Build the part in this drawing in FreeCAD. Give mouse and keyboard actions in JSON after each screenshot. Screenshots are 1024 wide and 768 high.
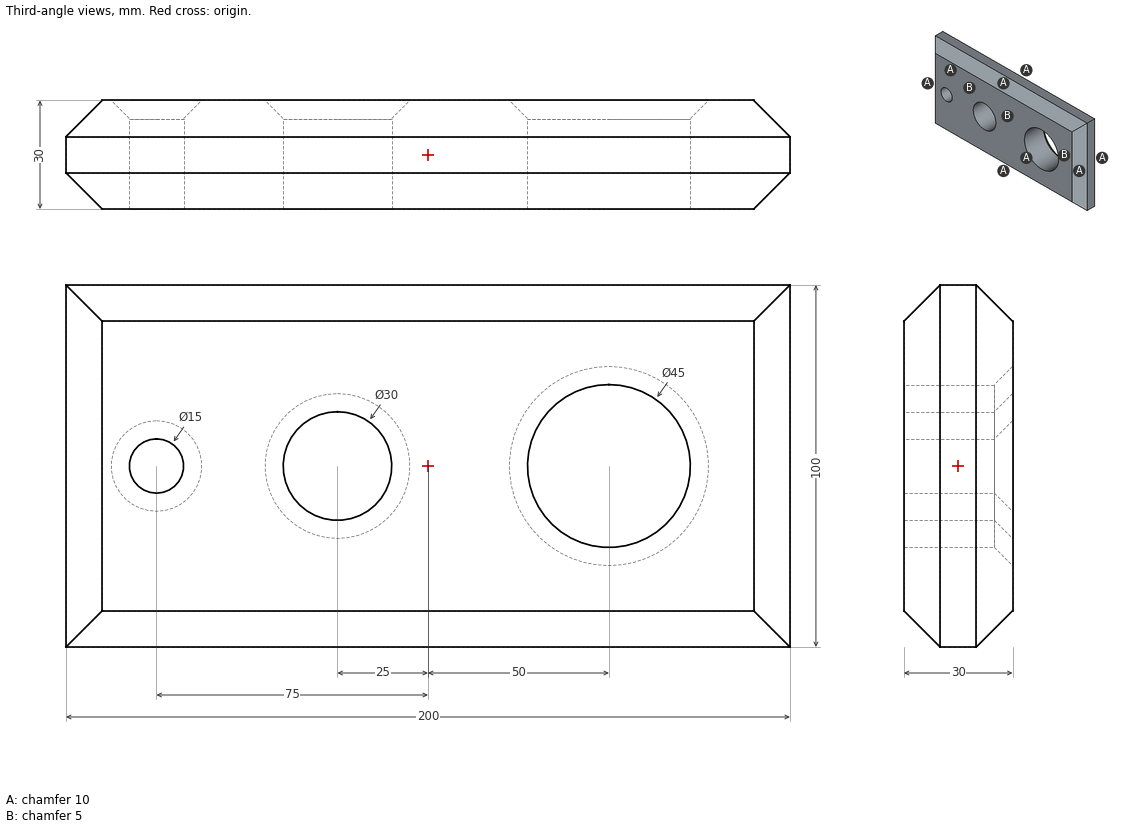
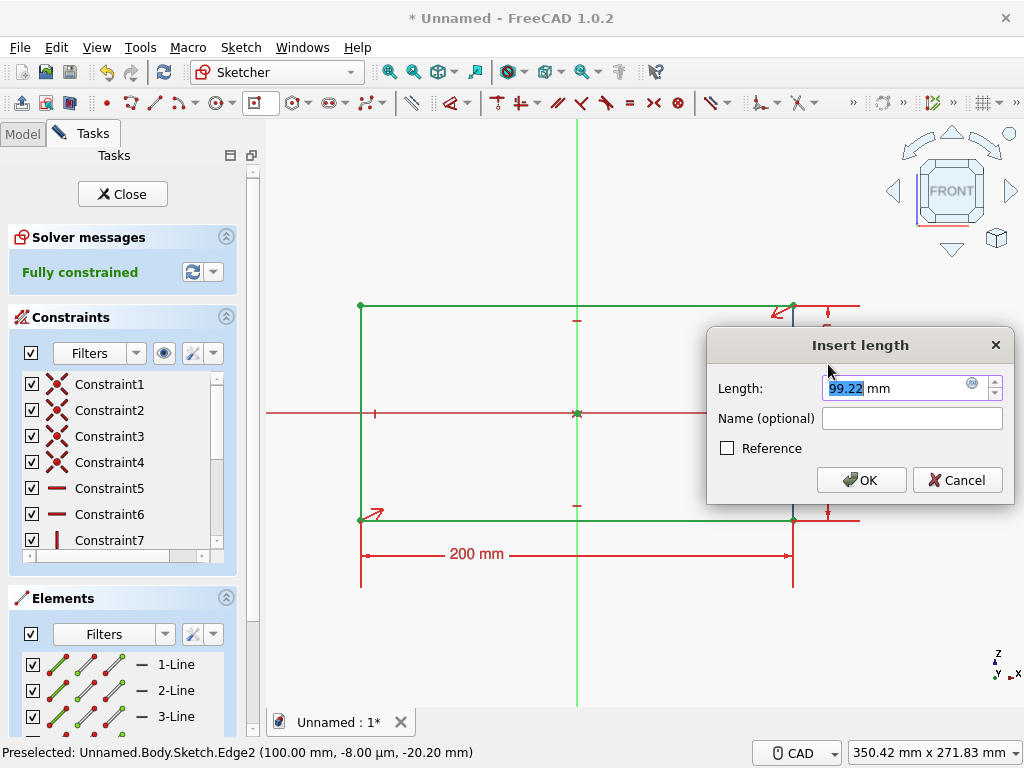
{"action": "type", "text": "100"}
{"action": "key", "text": "Return"}
{"action": "key", "text": "Escape"}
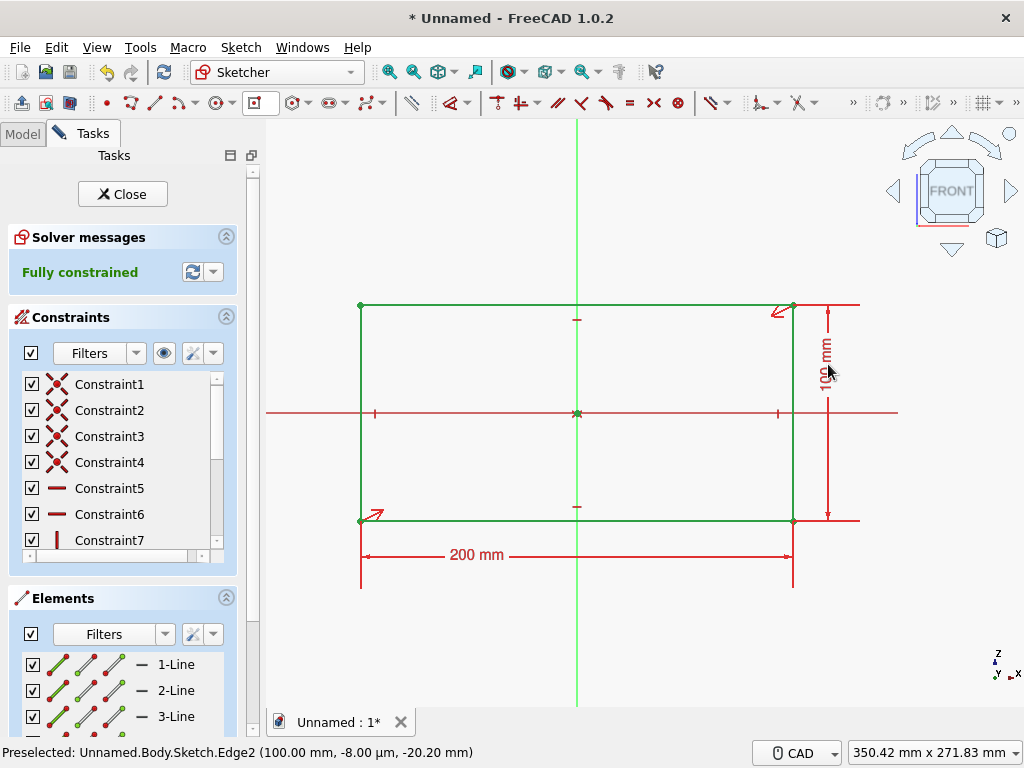
{"action": "left_click", "coordinate": [123, 194]}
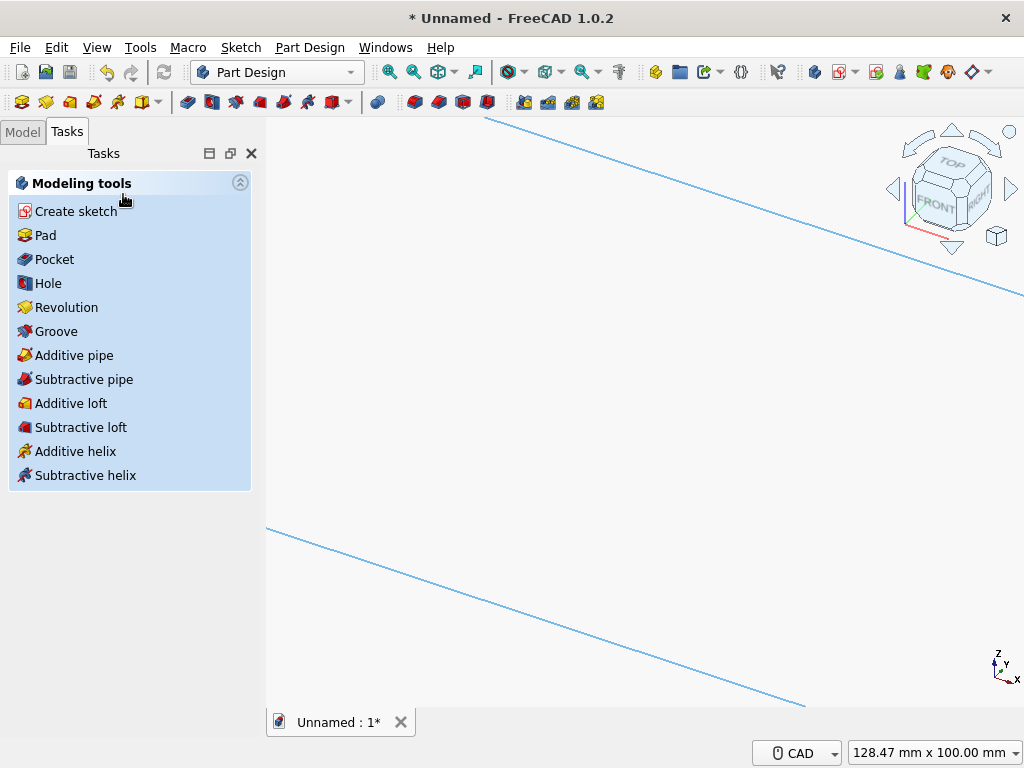
{"action": "left_click", "coordinate": [22, 102]}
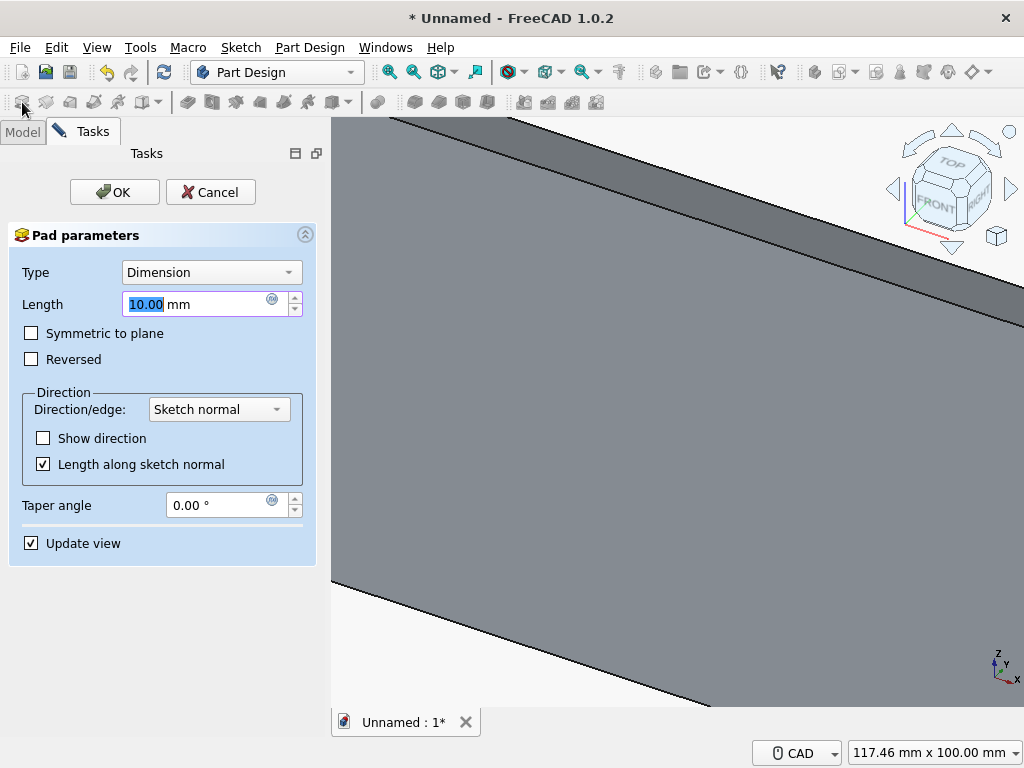
{"action": "type", "text": "30"}
{"action": "key", "text": "Tab"}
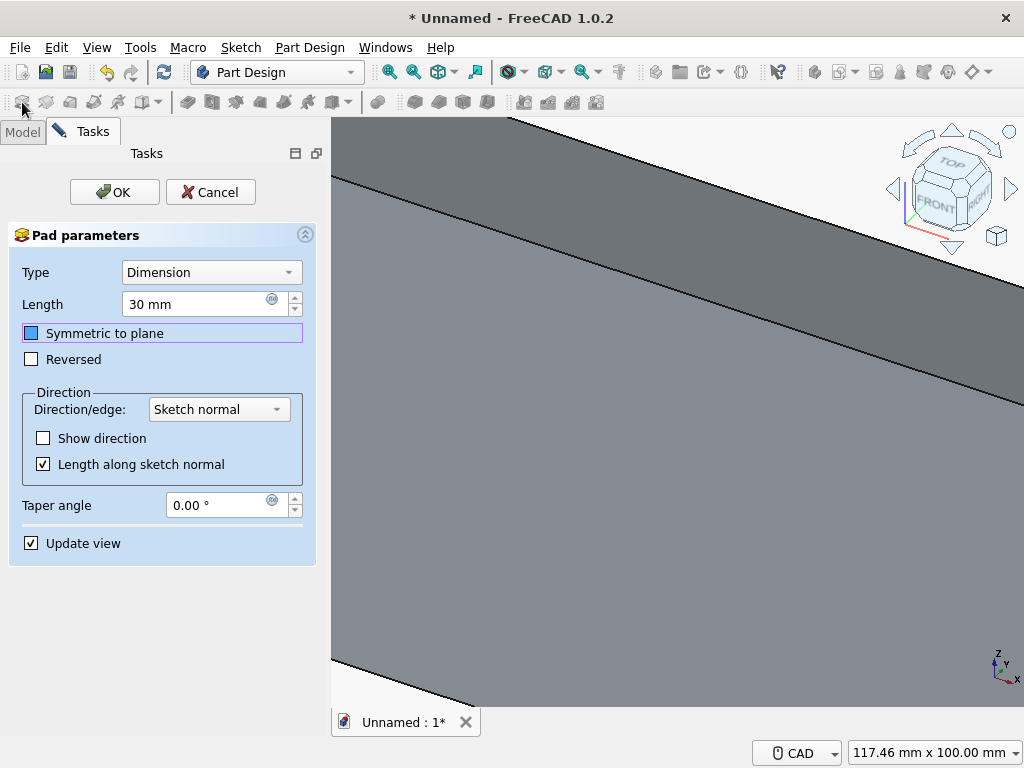
{"action": "left_click", "coordinate": [30, 333]}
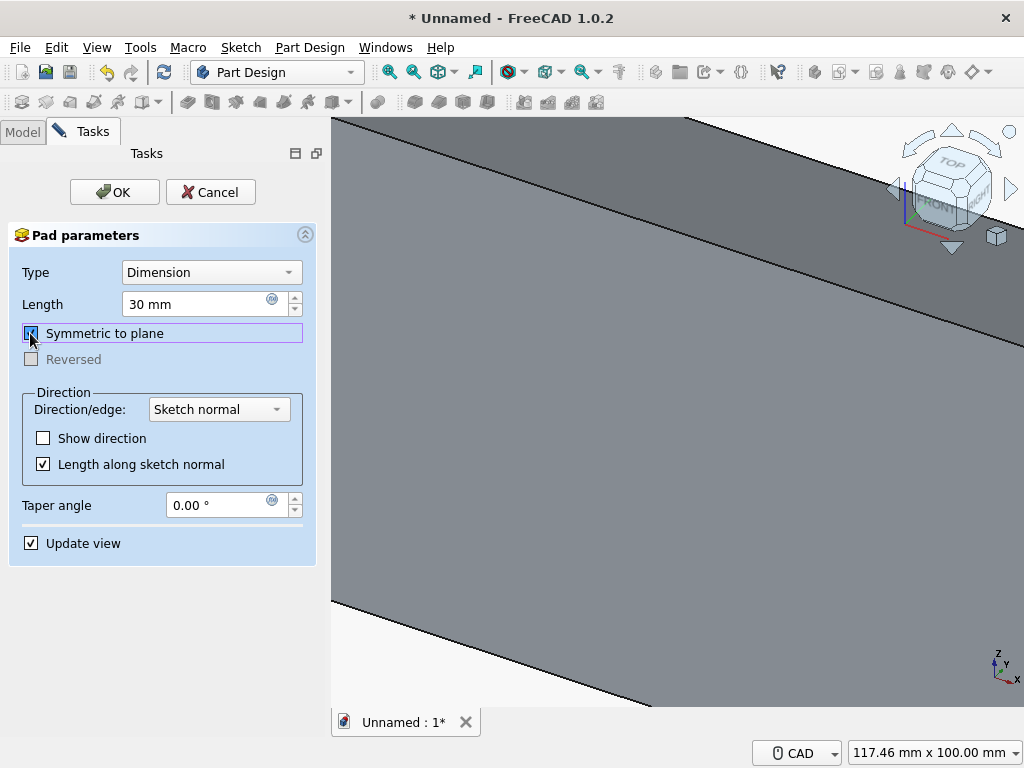
{"action": "left_click", "coordinate": [115, 192]}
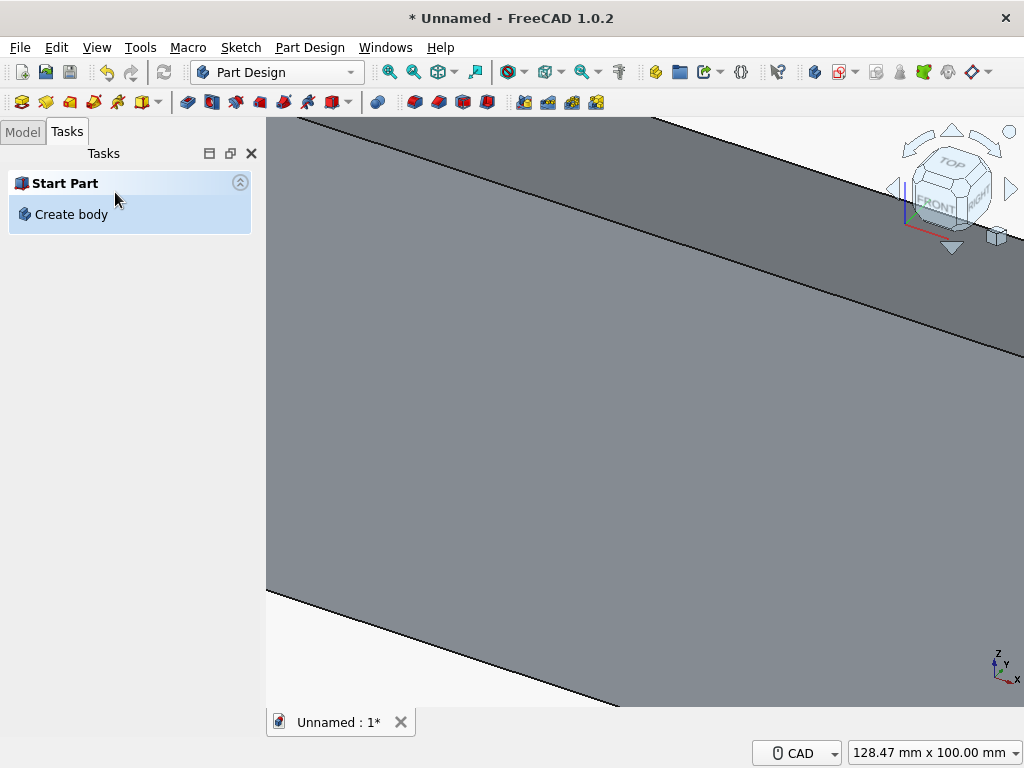
{"action": "left_click", "coordinate": [390, 72]}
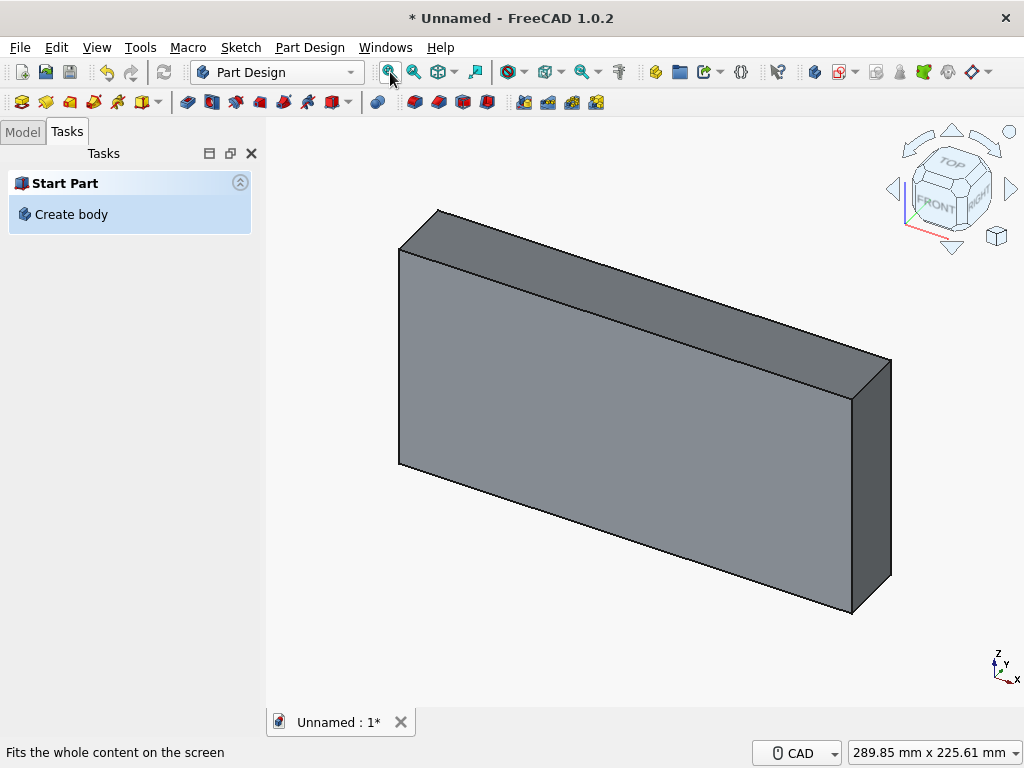
{"action": "left_click", "coordinate": [690, 452]}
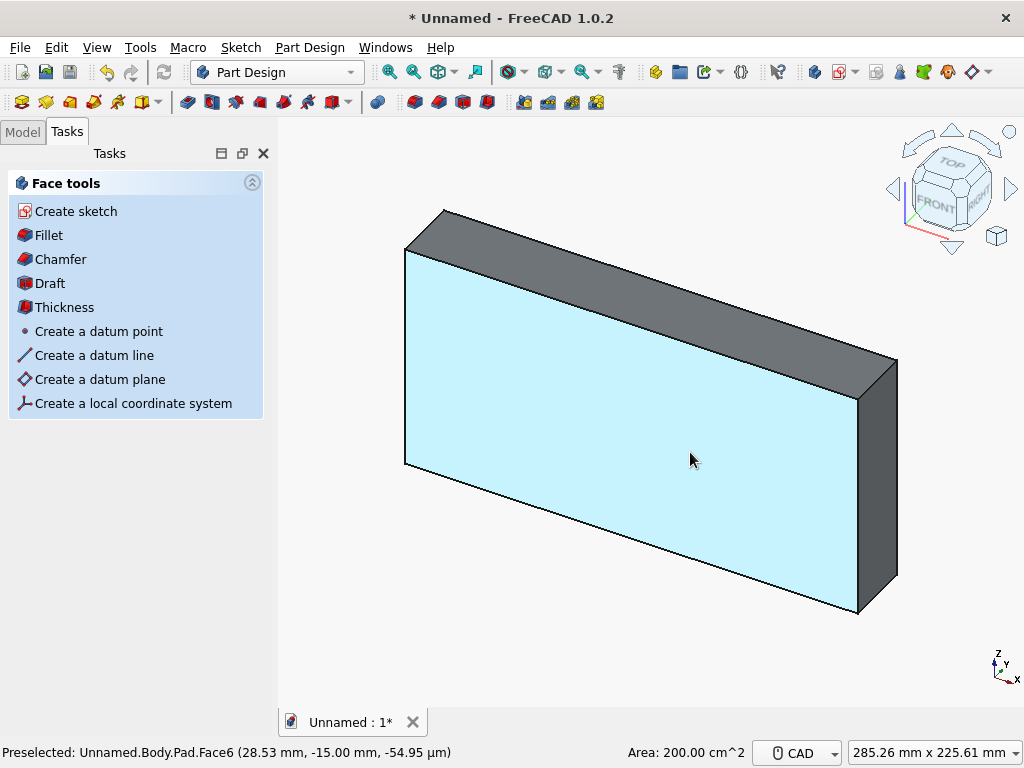
{"action": "key", "text": "0"}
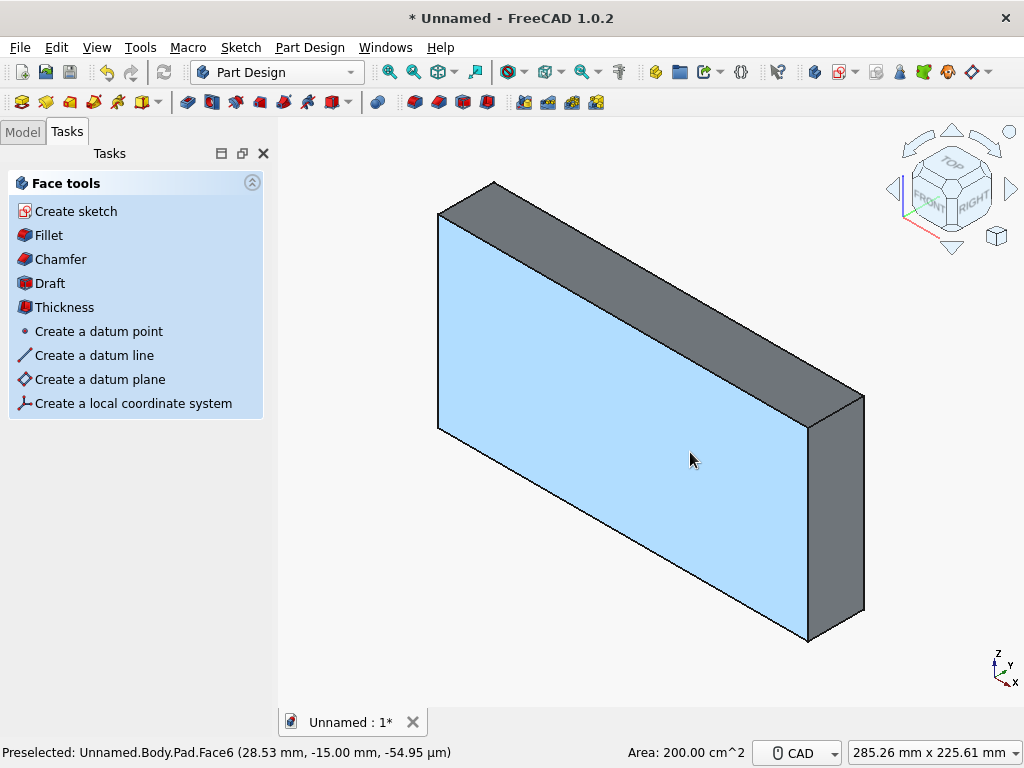
{"action": "key", "text": "2"}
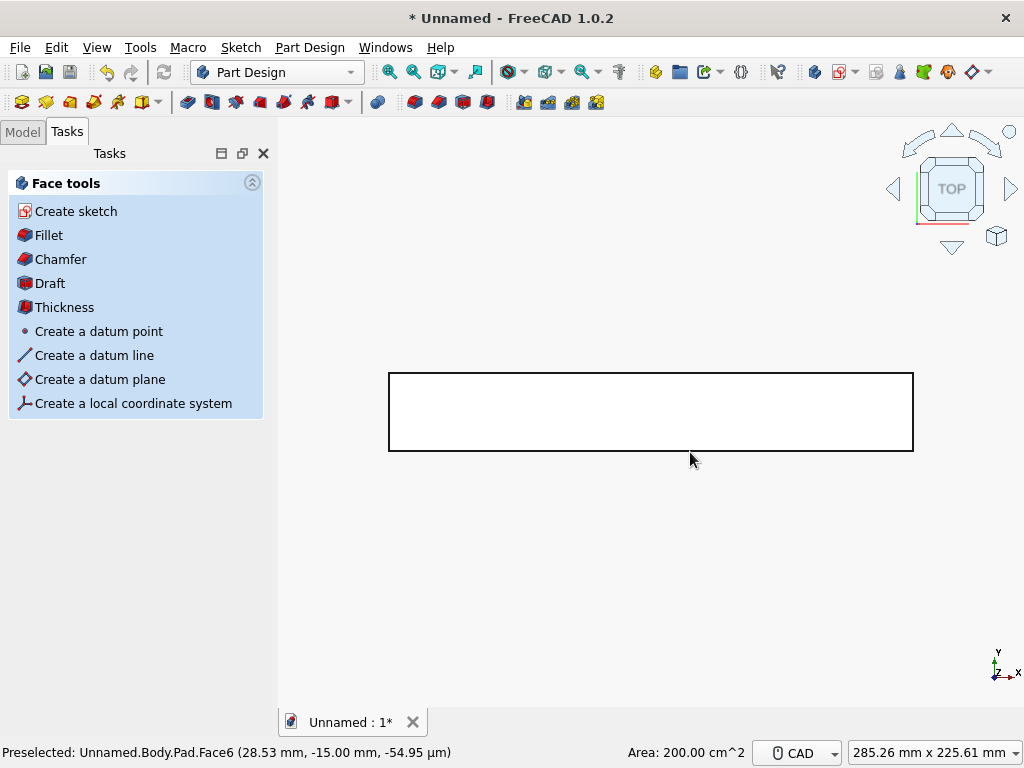
{"action": "key", "text": "1"}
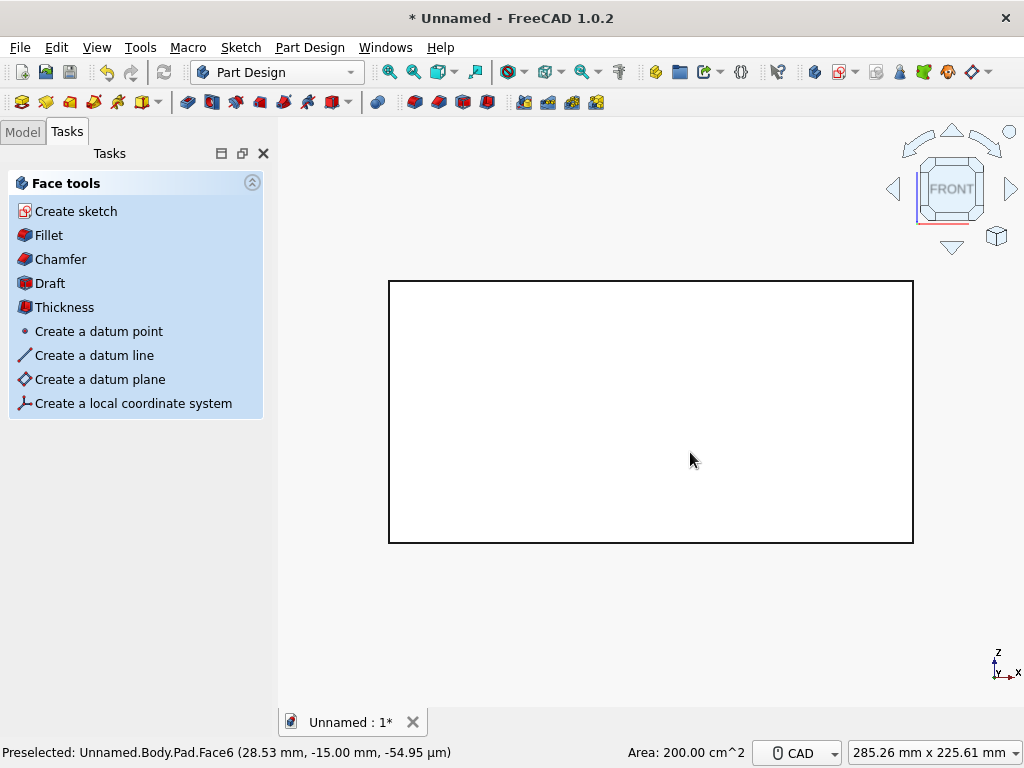
{"action": "key", "text": "3"}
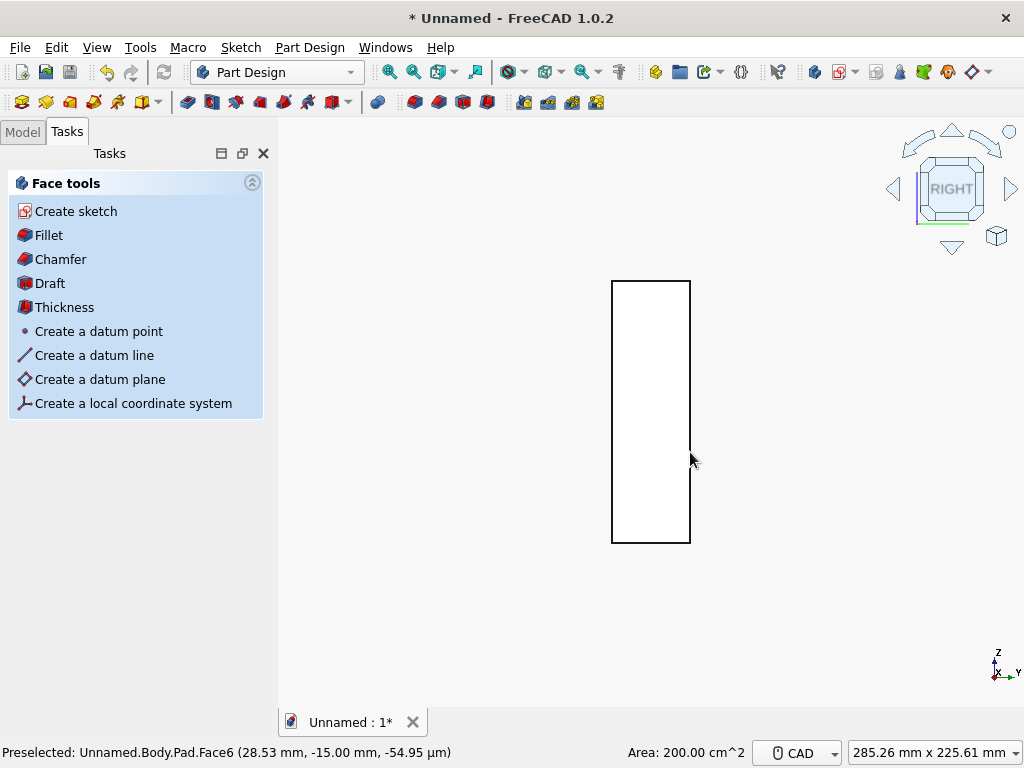
{"action": "left_click", "coordinate": [390, 72]}